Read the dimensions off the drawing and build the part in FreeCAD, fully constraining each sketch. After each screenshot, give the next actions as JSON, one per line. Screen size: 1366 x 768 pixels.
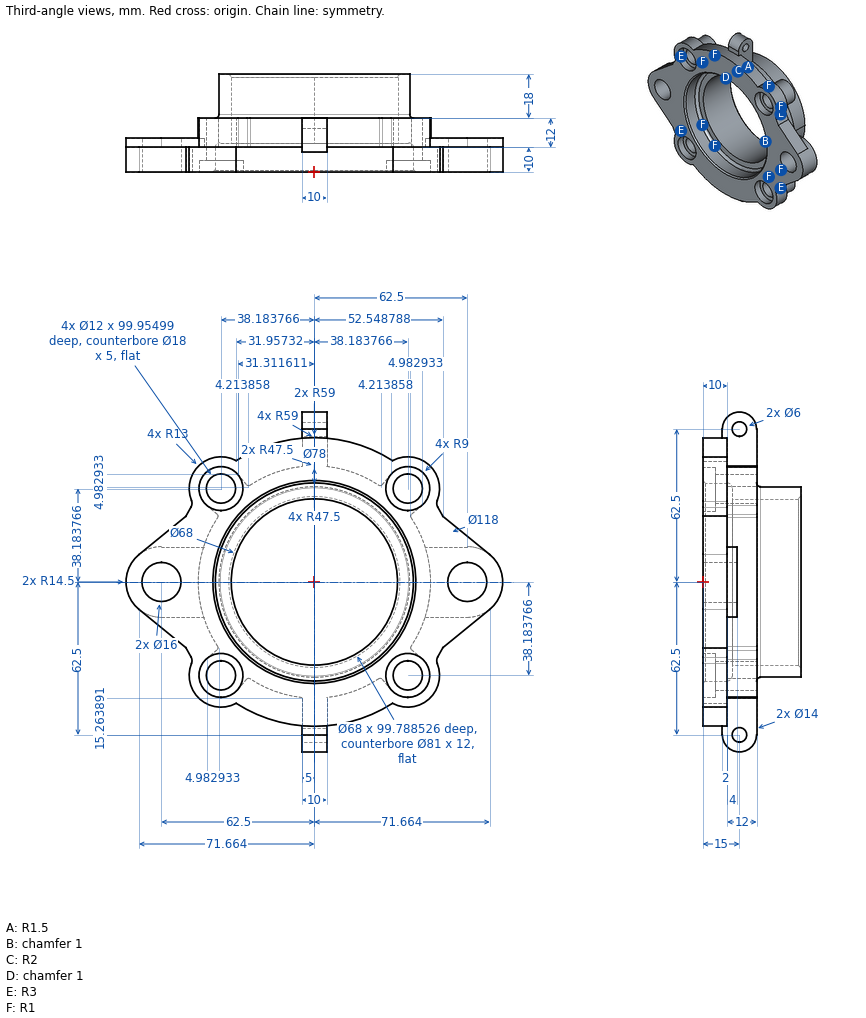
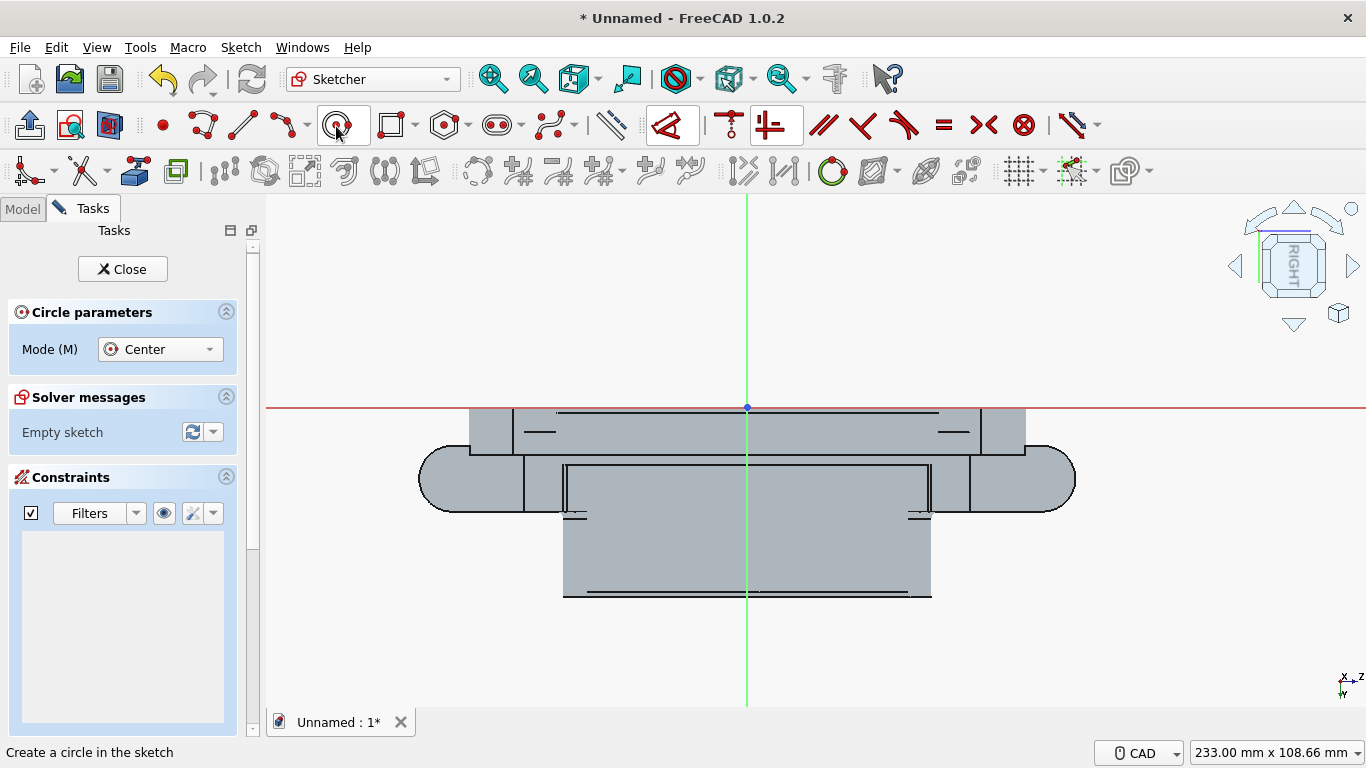
{"action": "scroll", "coordinate": [1042, 479], "scroll_direction": "up", "scroll_amount": 3}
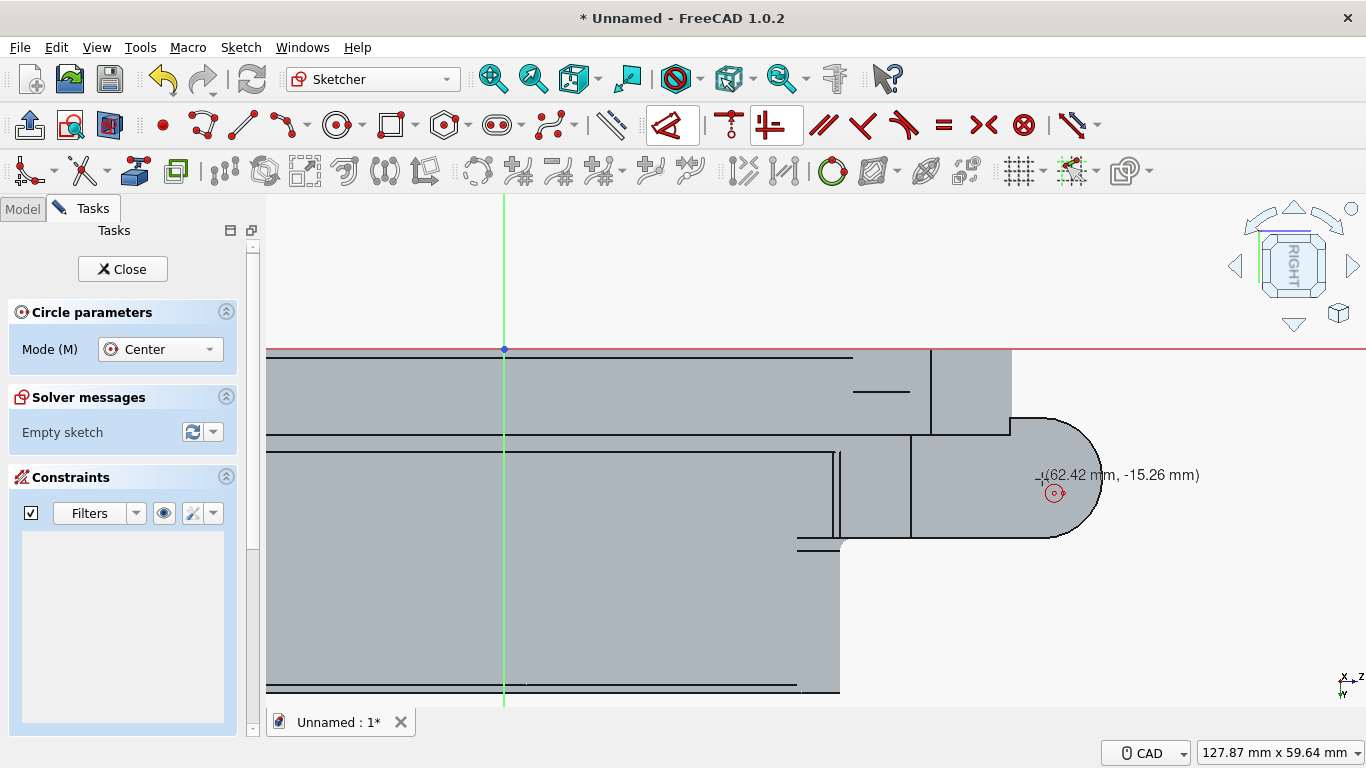
{"action": "left_click", "coordinate": [1042, 478]}
{"action": "left_click", "coordinate": [1060, 460]}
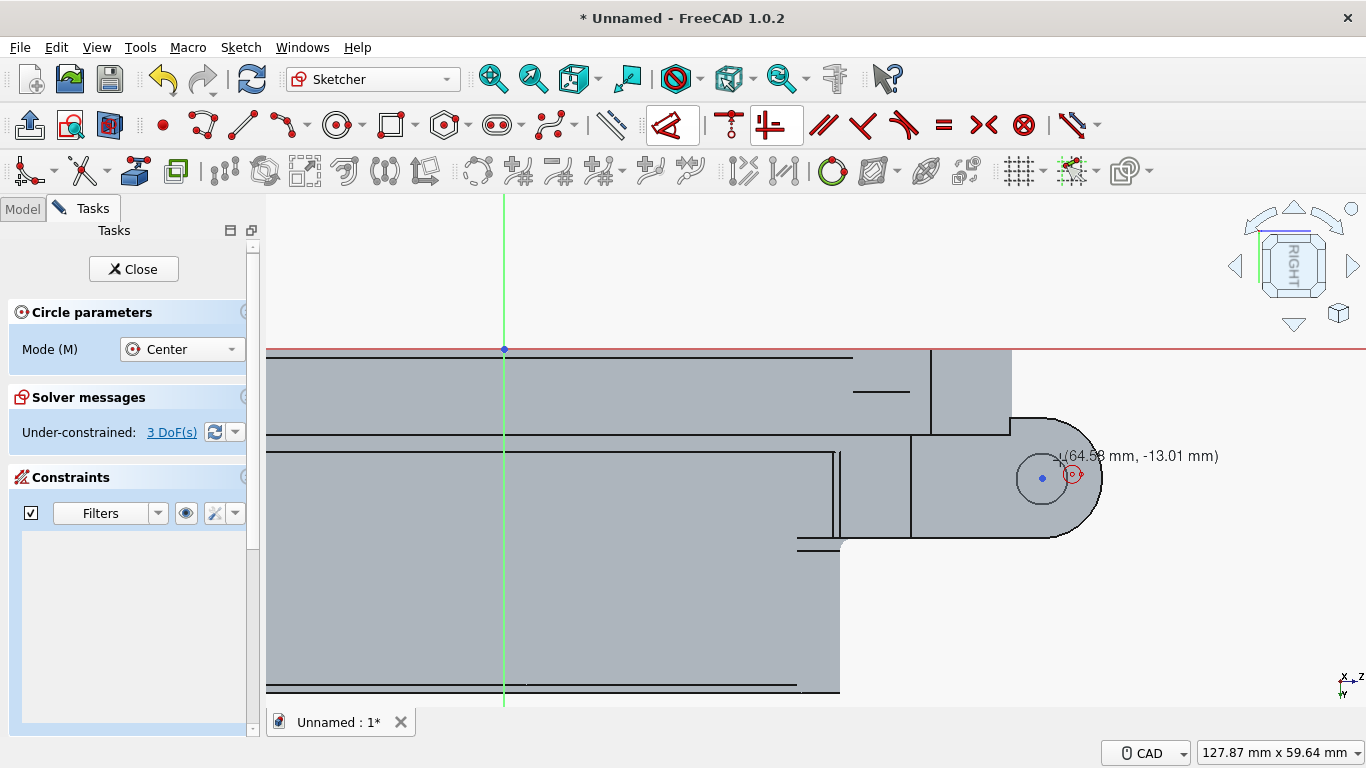
{"action": "scroll", "coordinate": [1043, 480], "scroll_direction": "down", "scroll_amount": 3}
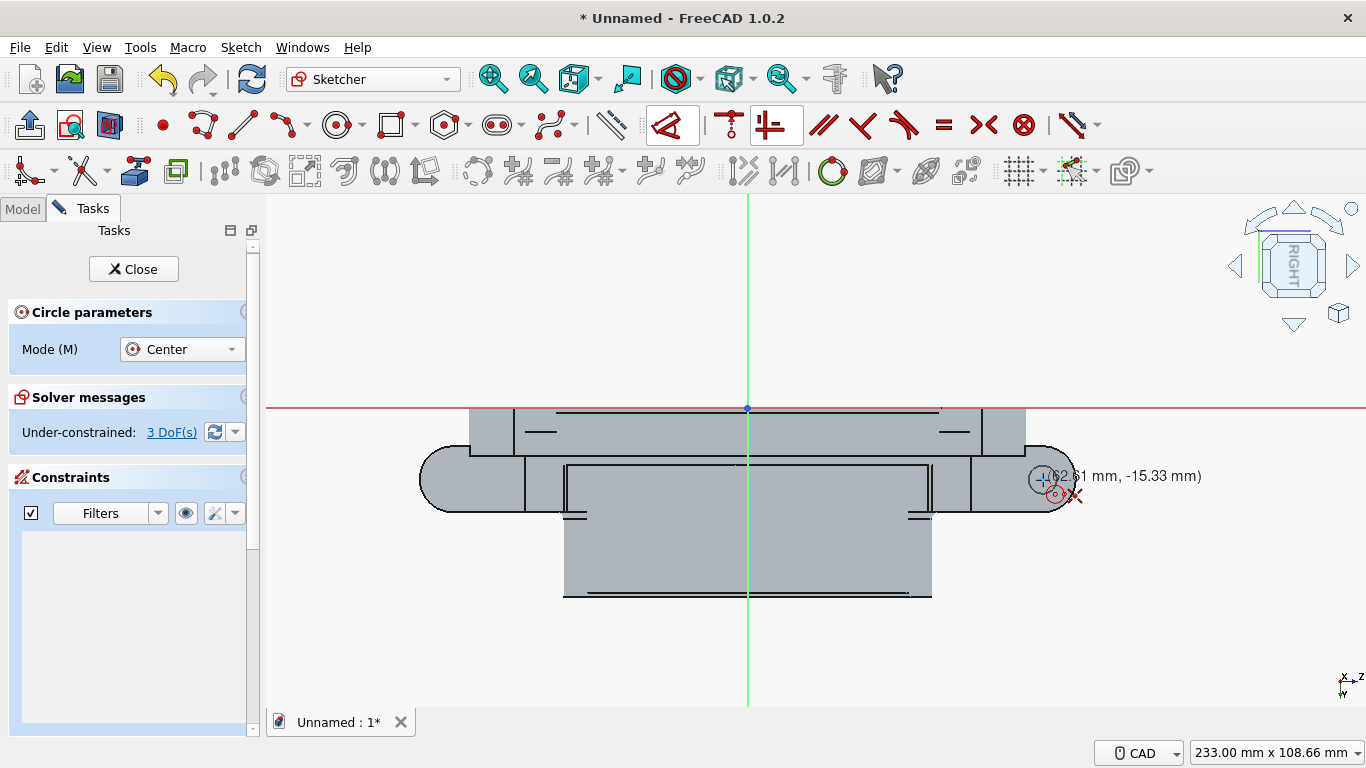
{"action": "scroll", "coordinate": [453, 479], "scroll_direction": "up", "scroll_amount": 3}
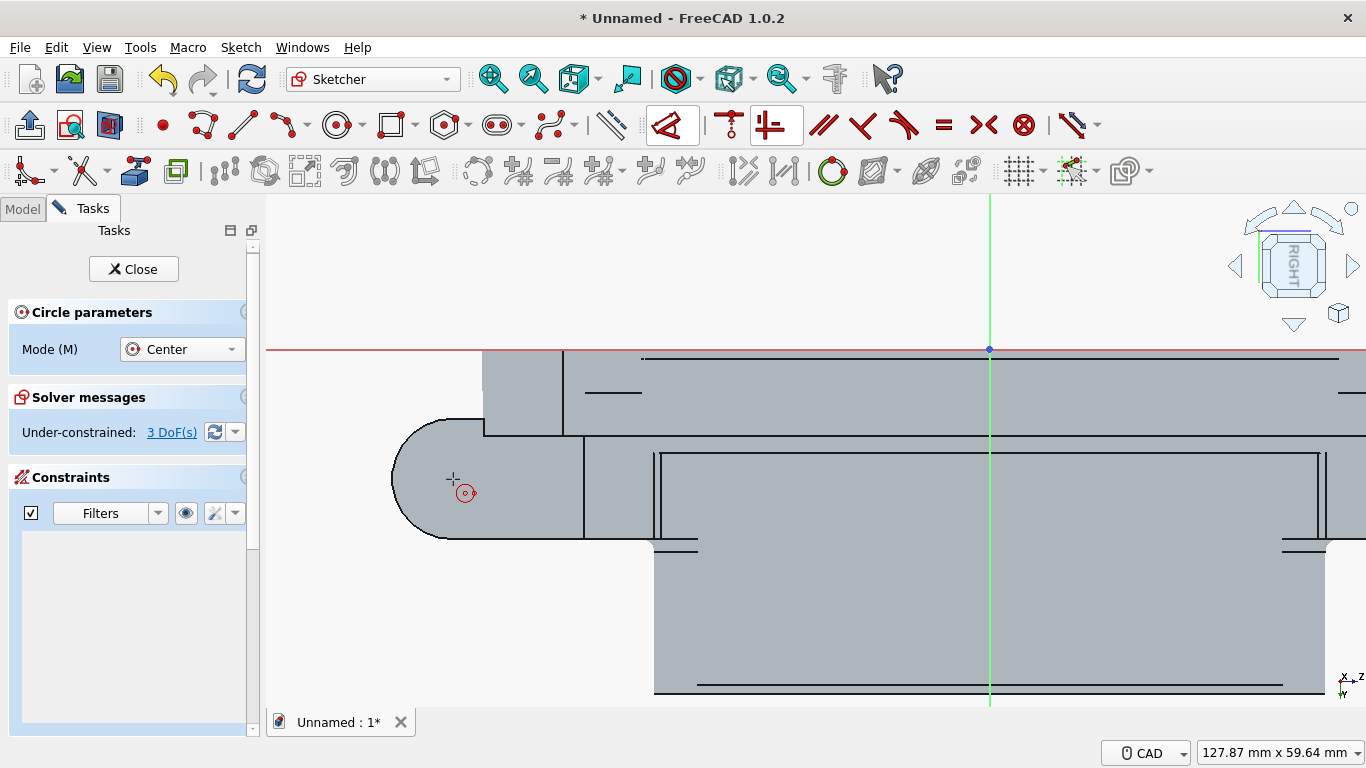
{"action": "left_click", "coordinate": [452, 479]}
{"action": "left_click", "coordinate": [471, 461]}
{"action": "key", "text": "Escape"}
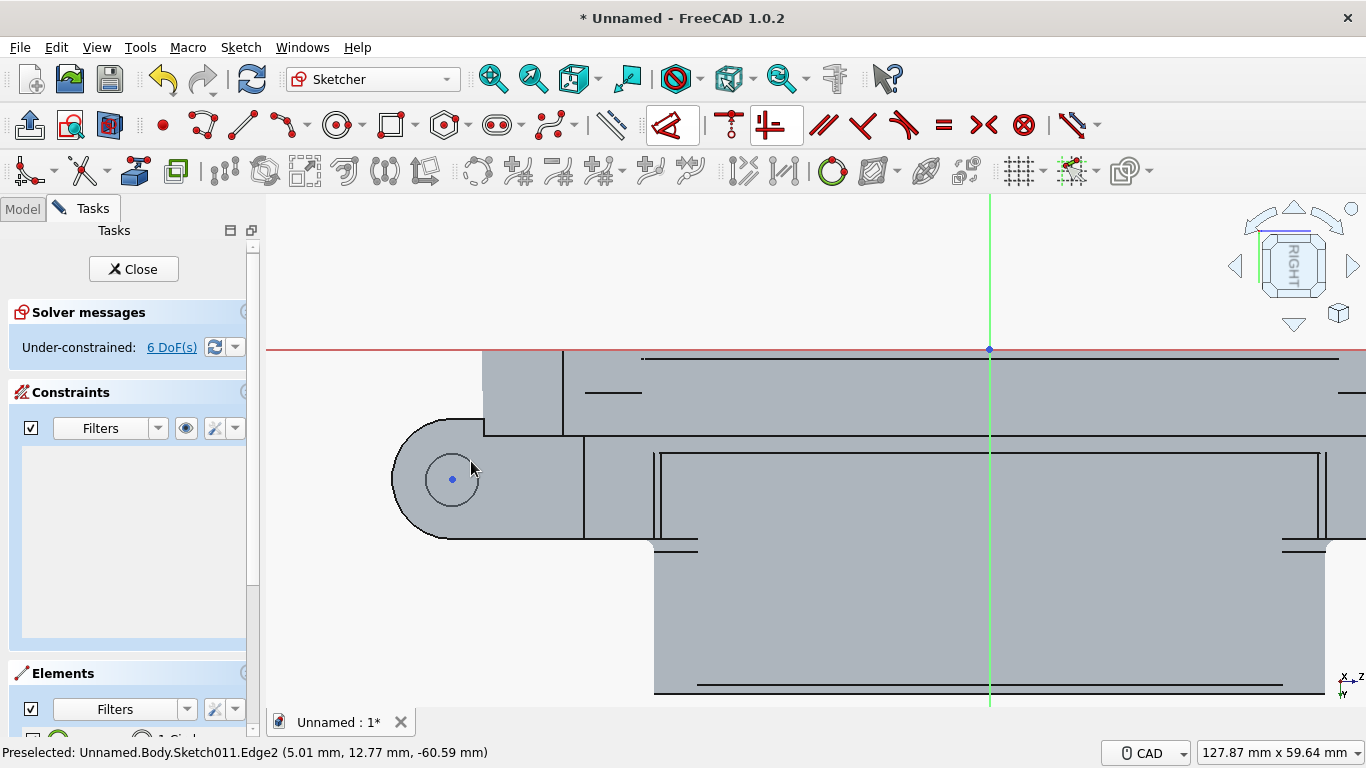
{"action": "scroll", "coordinate": [453, 479], "scroll_direction": "down", "scroll_amount": 3}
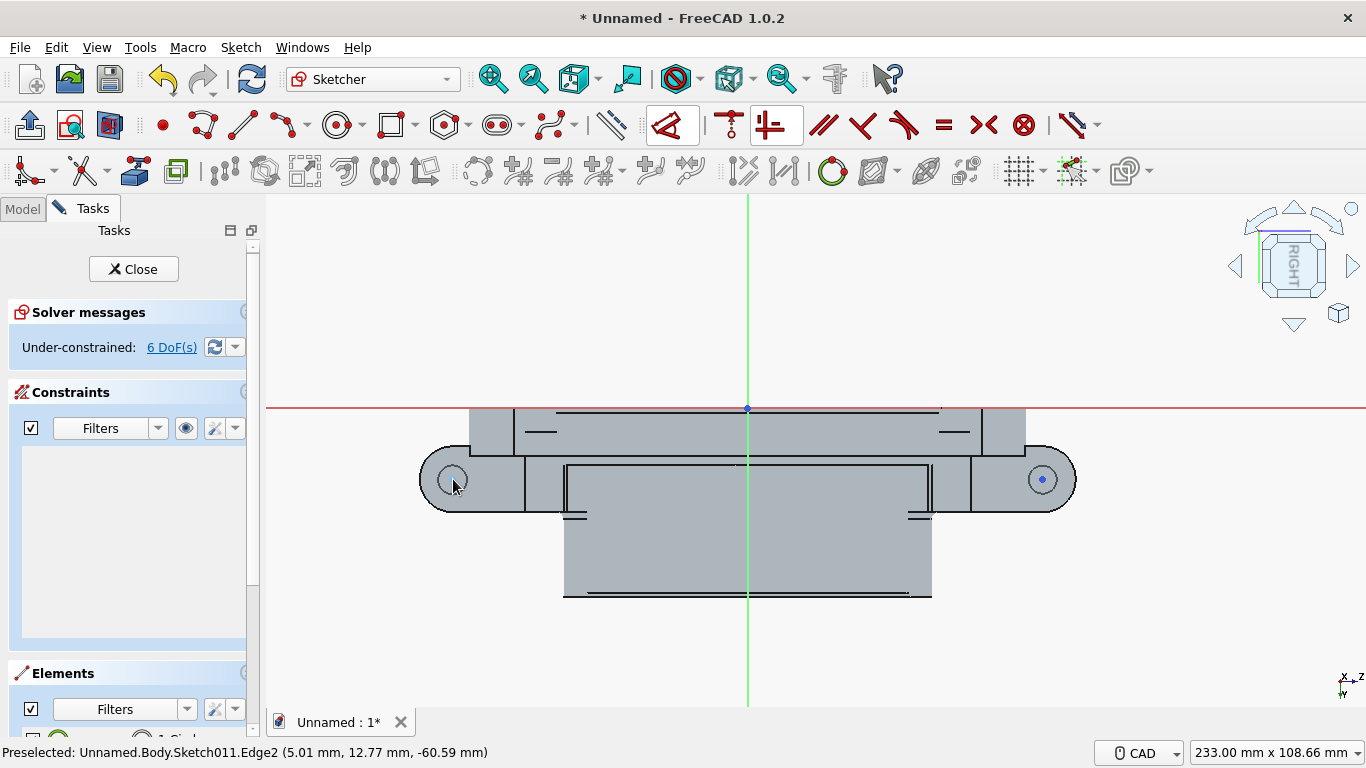
{"action": "left_click", "coordinate": [1053, 470]}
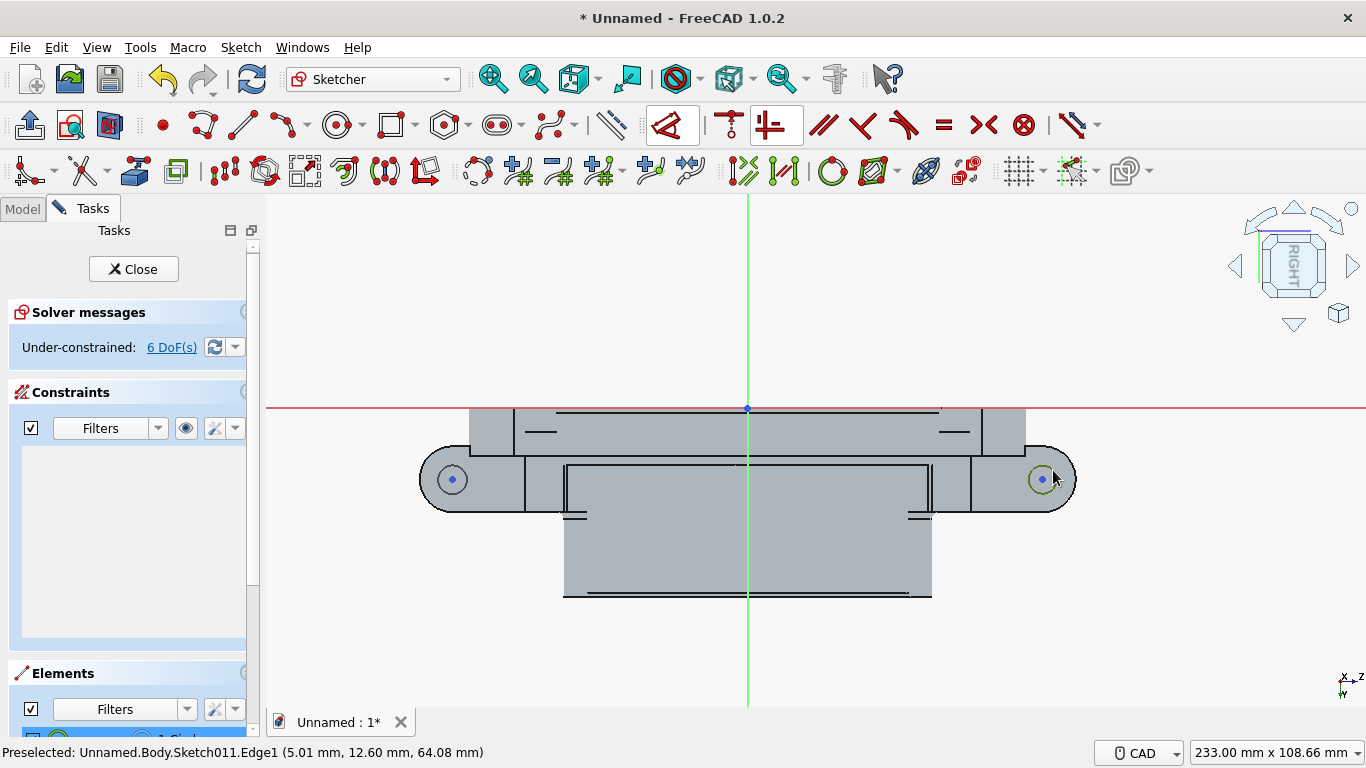
{"action": "left_click", "coordinate": [463, 470]}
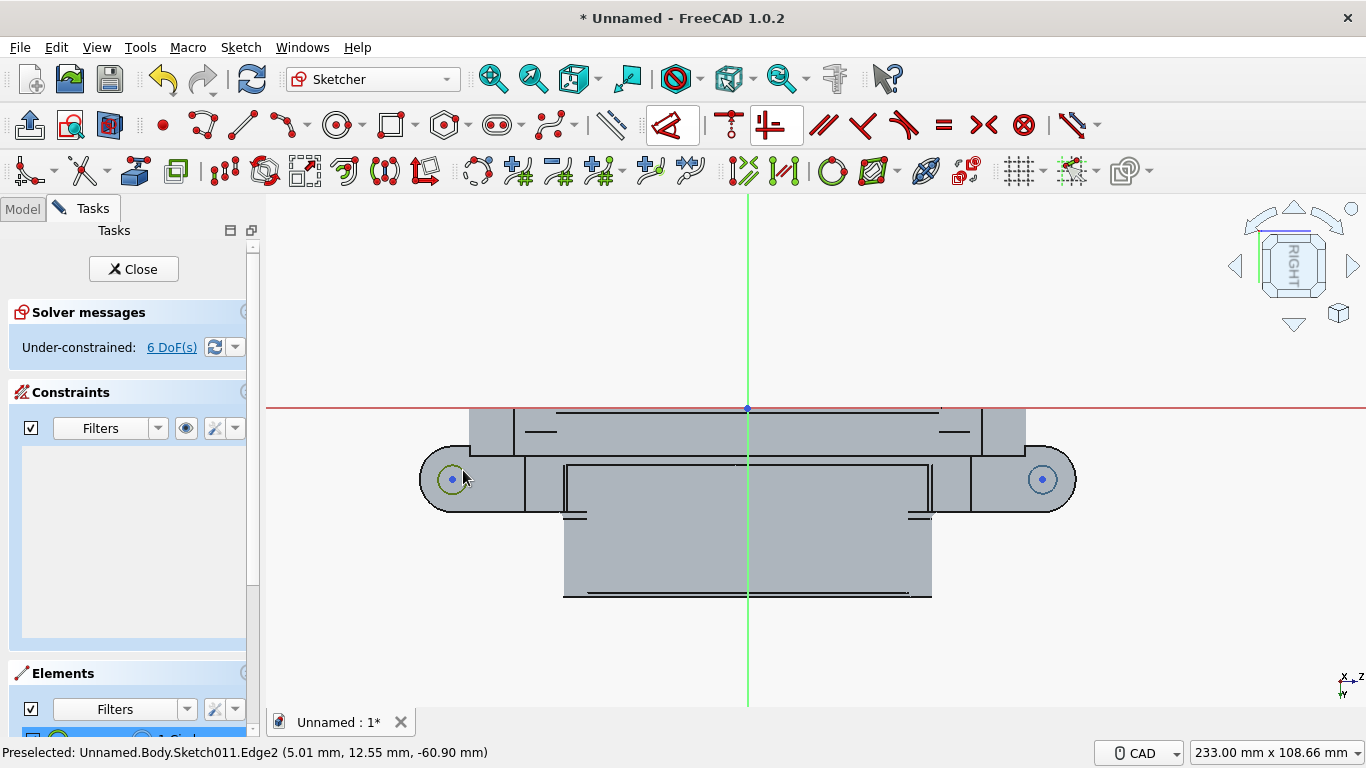
{"action": "left_click", "coordinate": [944, 126]}